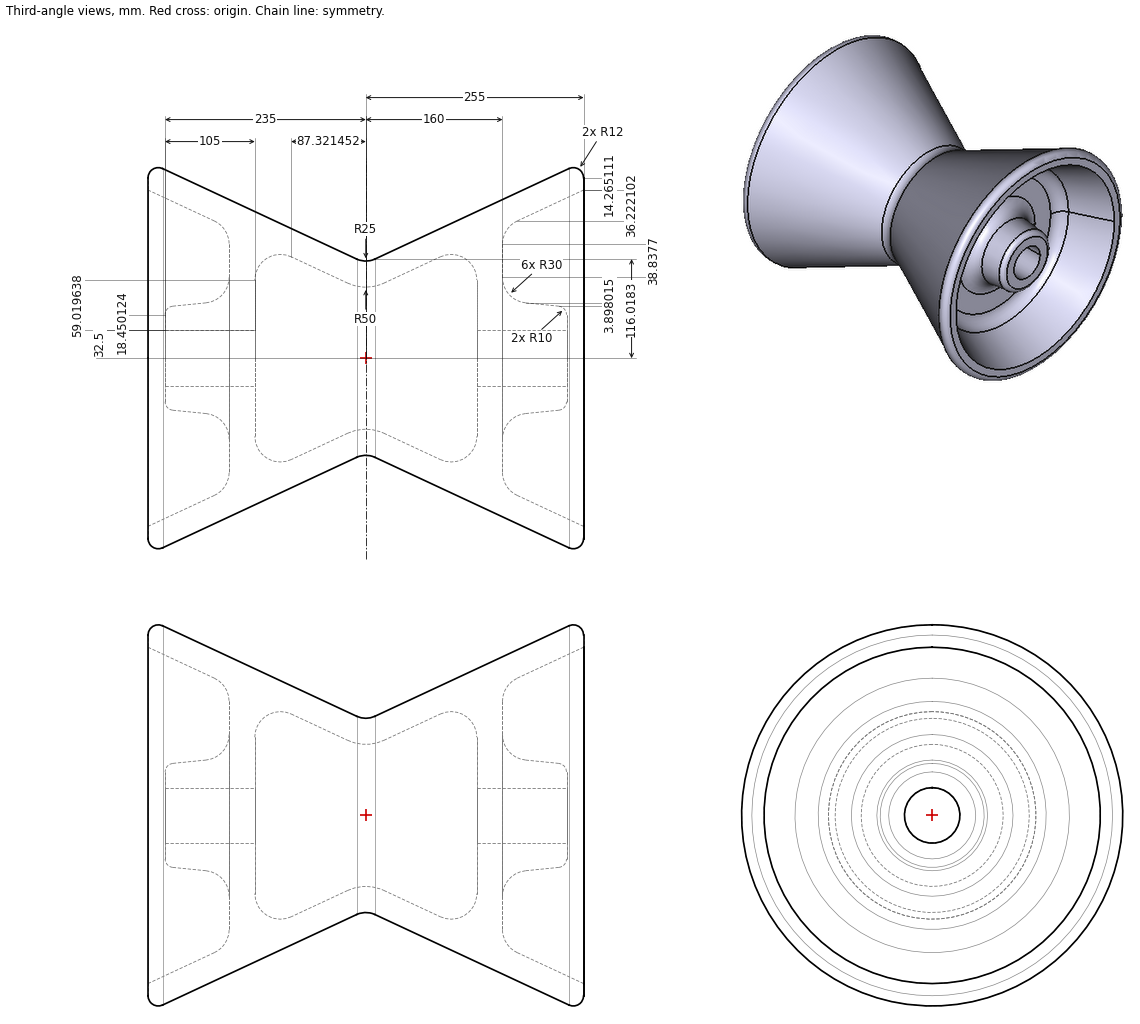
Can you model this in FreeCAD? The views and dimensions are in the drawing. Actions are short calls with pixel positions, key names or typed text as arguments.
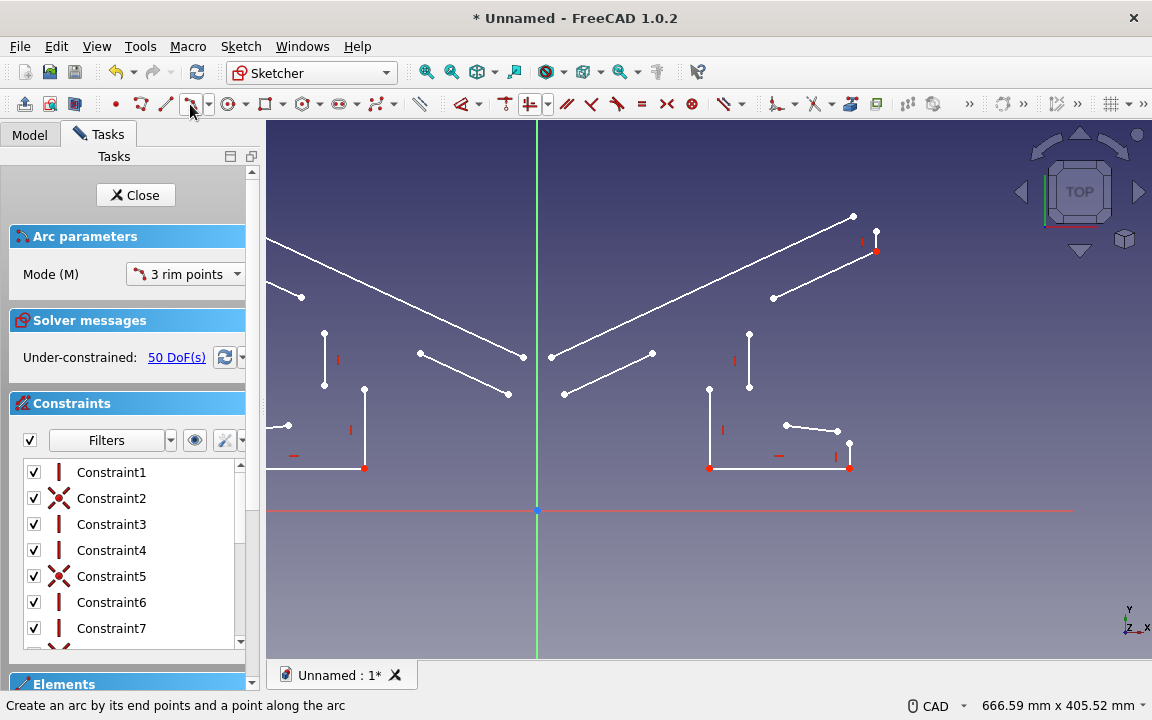
click(787, 426)
click(749, 387)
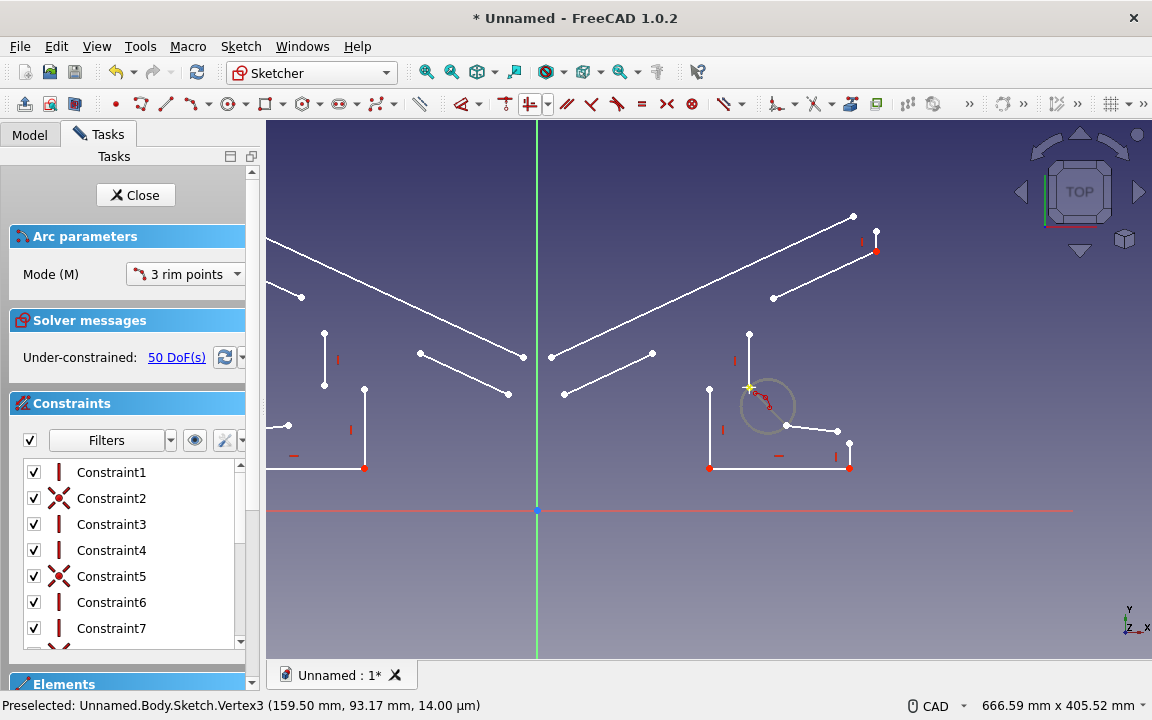
scroll(760, 412, up, 3)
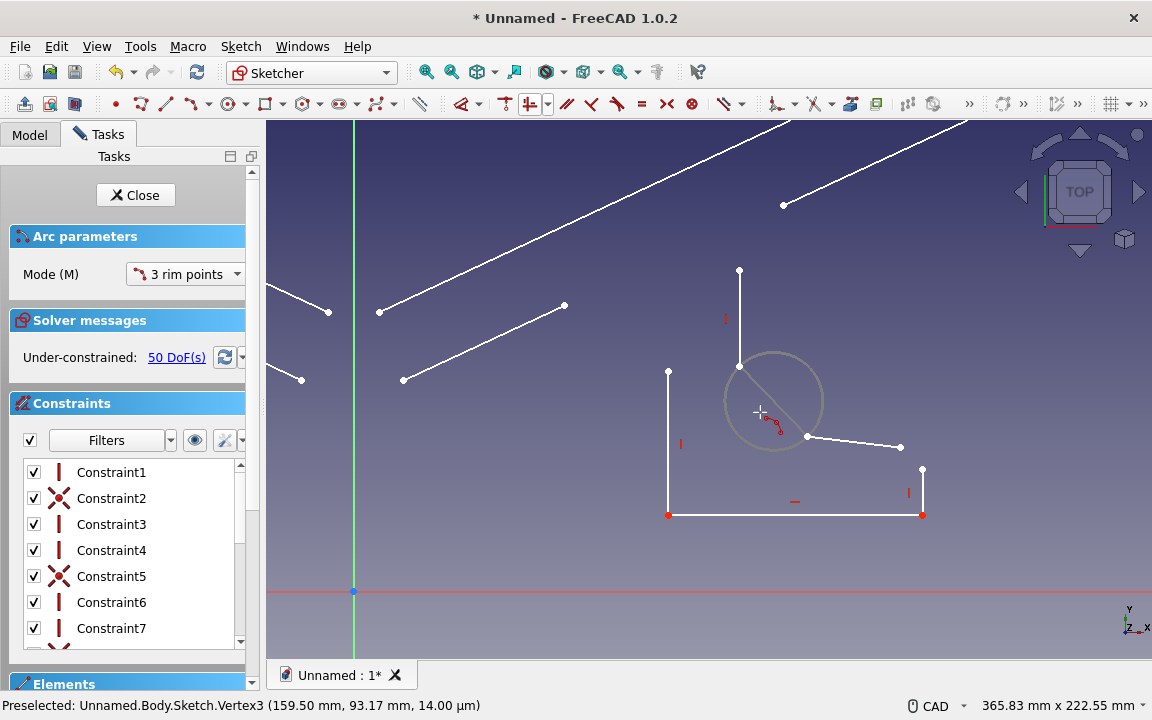
click(760, 411)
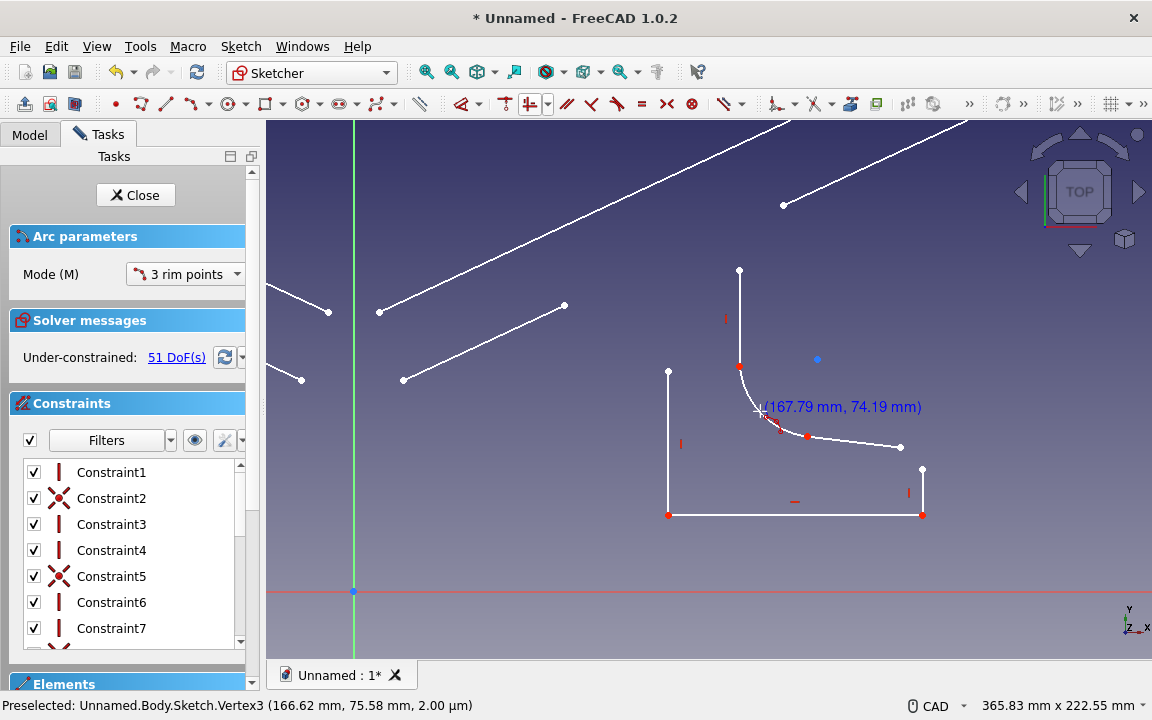
click(740, 271)
click(783, 206)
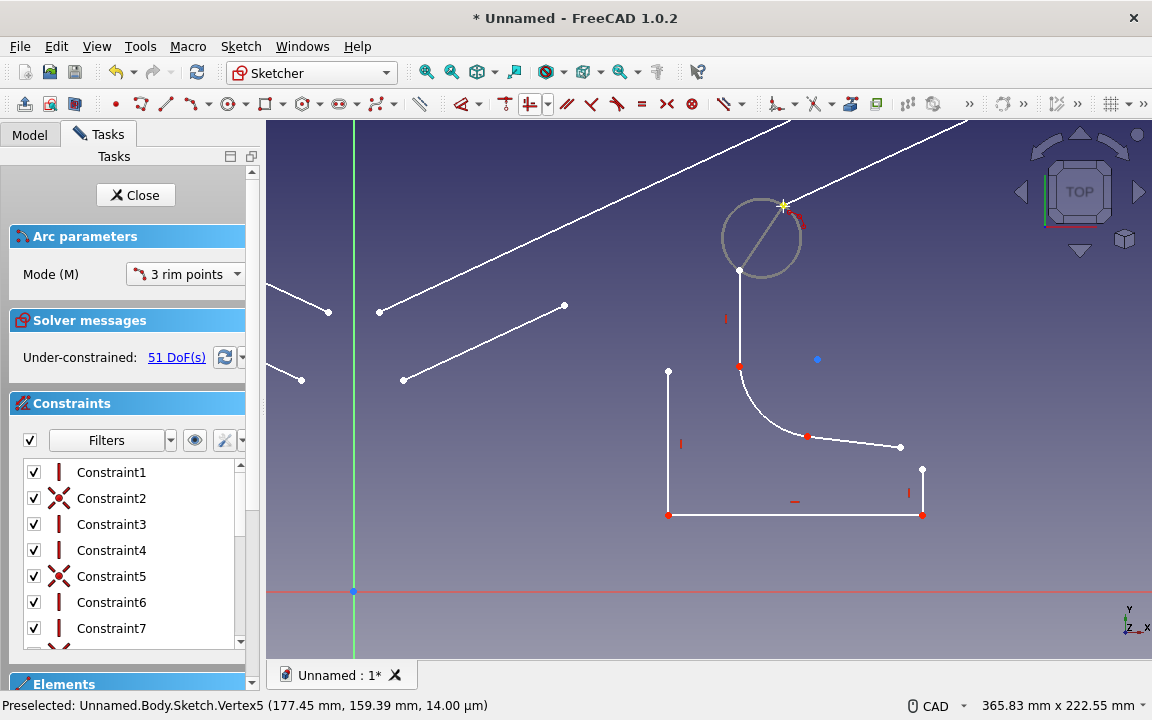
scroll(753, 229, up, 2)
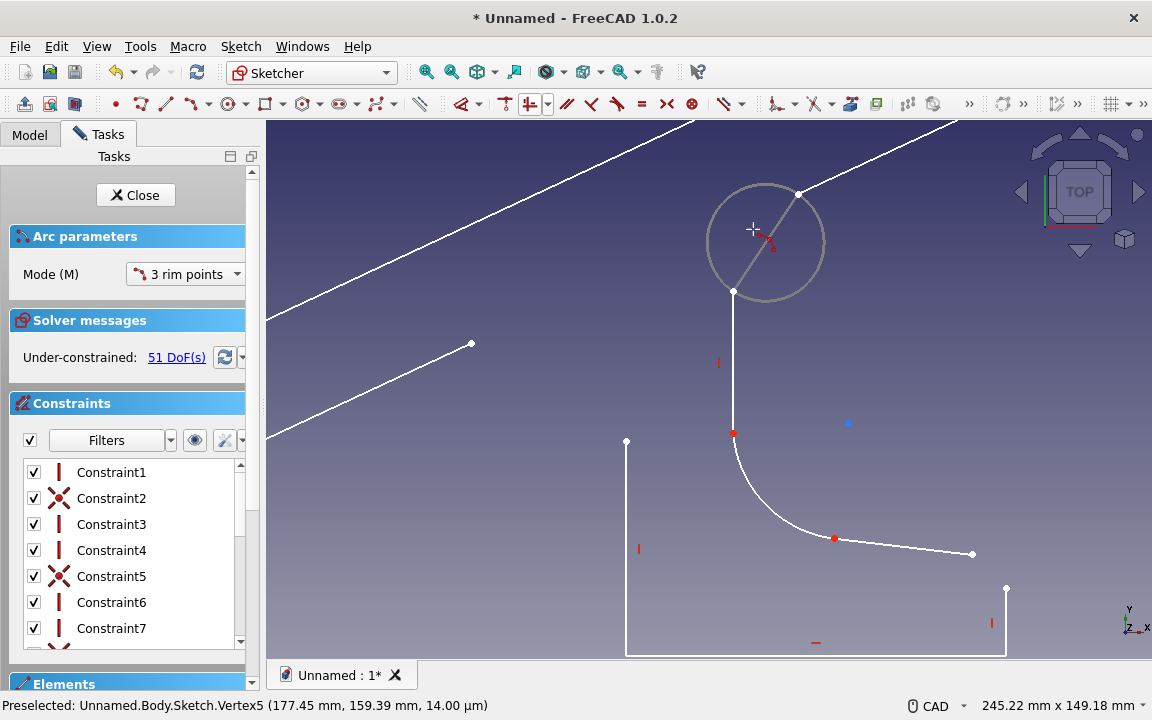
click(752, 229)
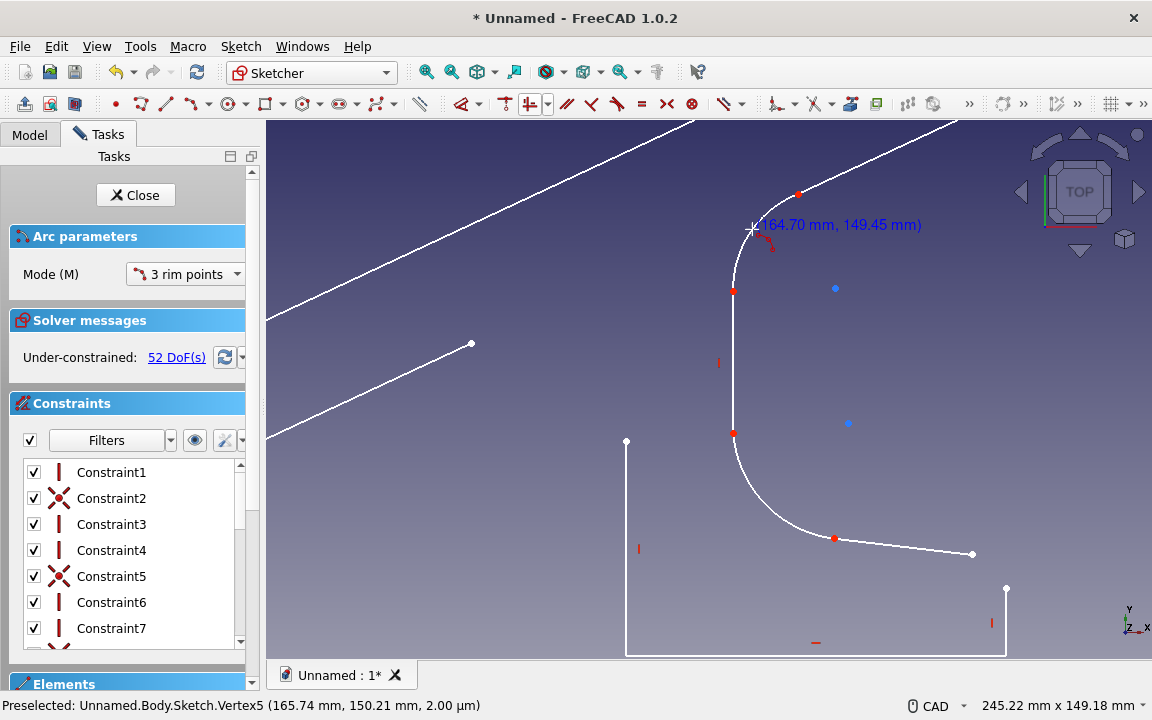
scroll(799, 396, down, 7)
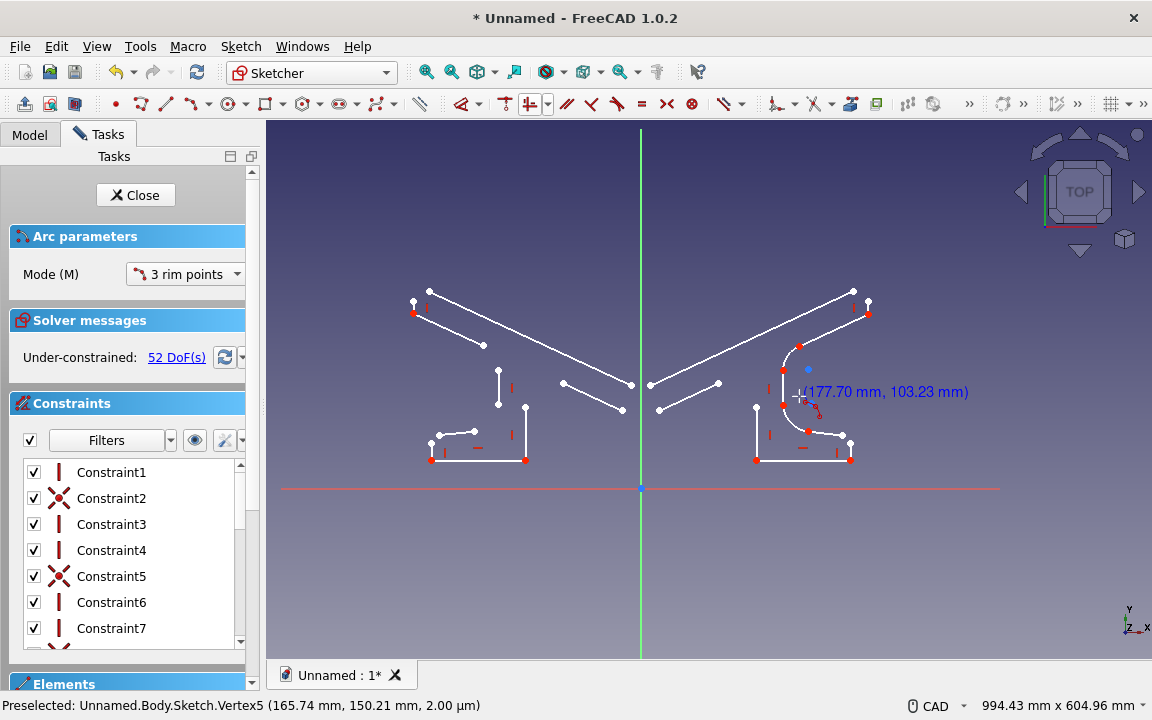
scroll(868, 300, up, 5)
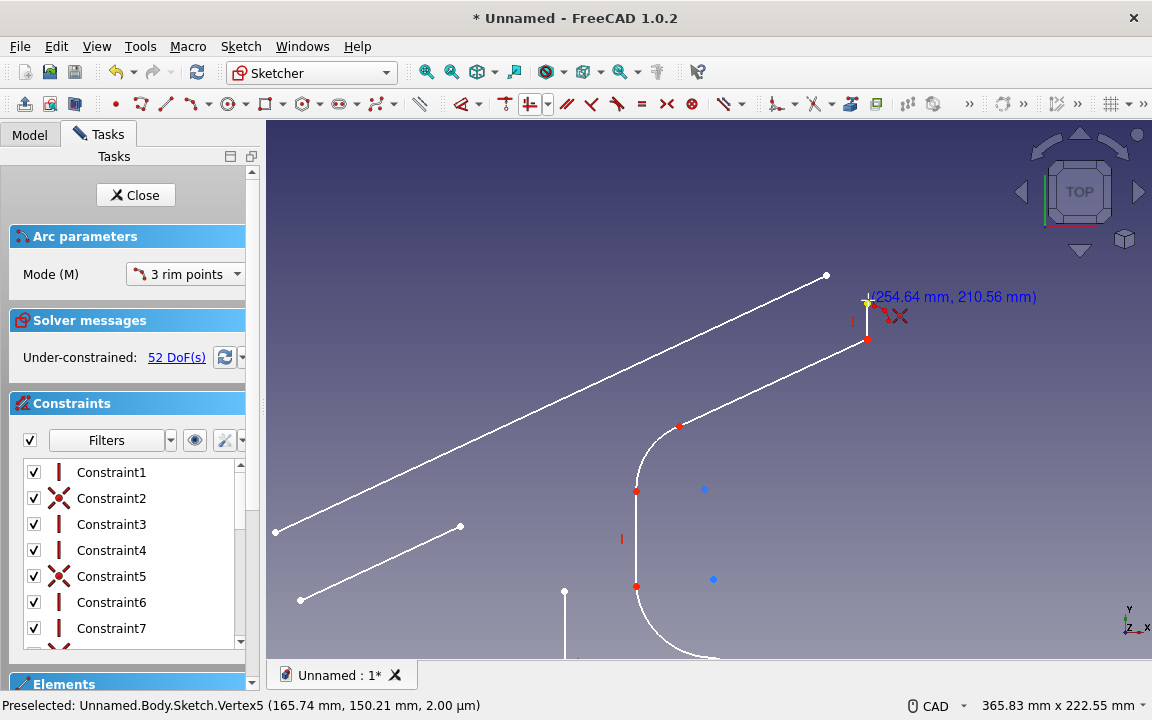
click(867, 303)
click(826, 276)
click(854, 276)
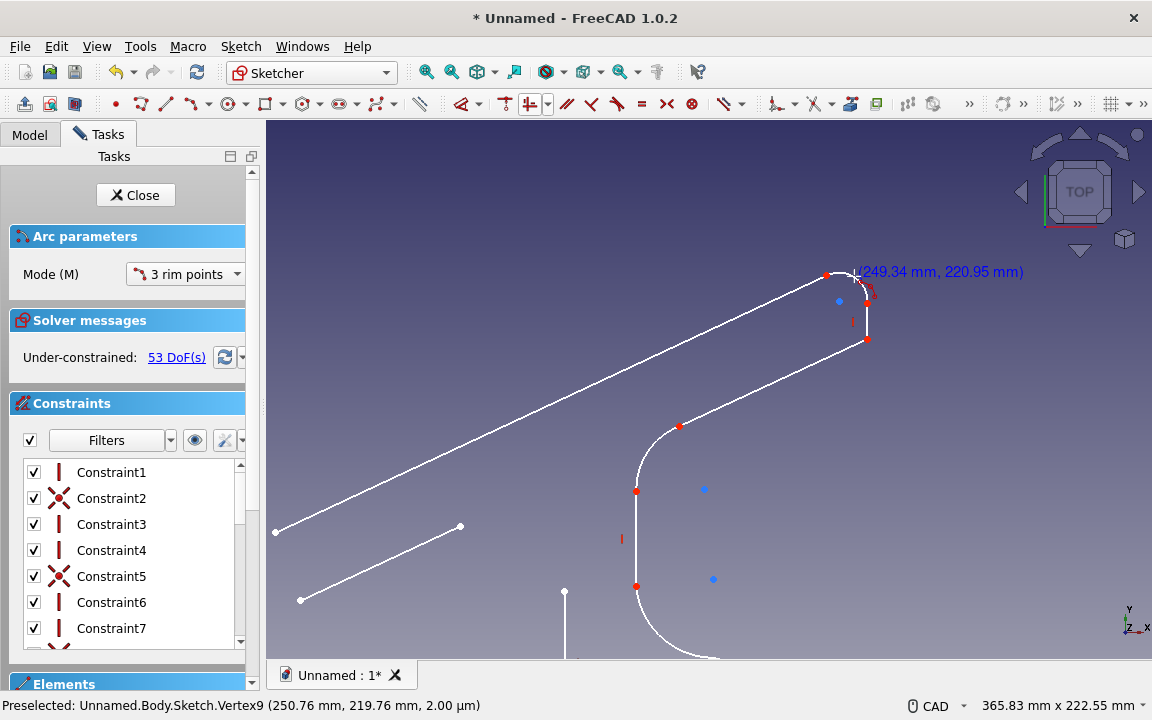
scroll(868, 300, down, 5)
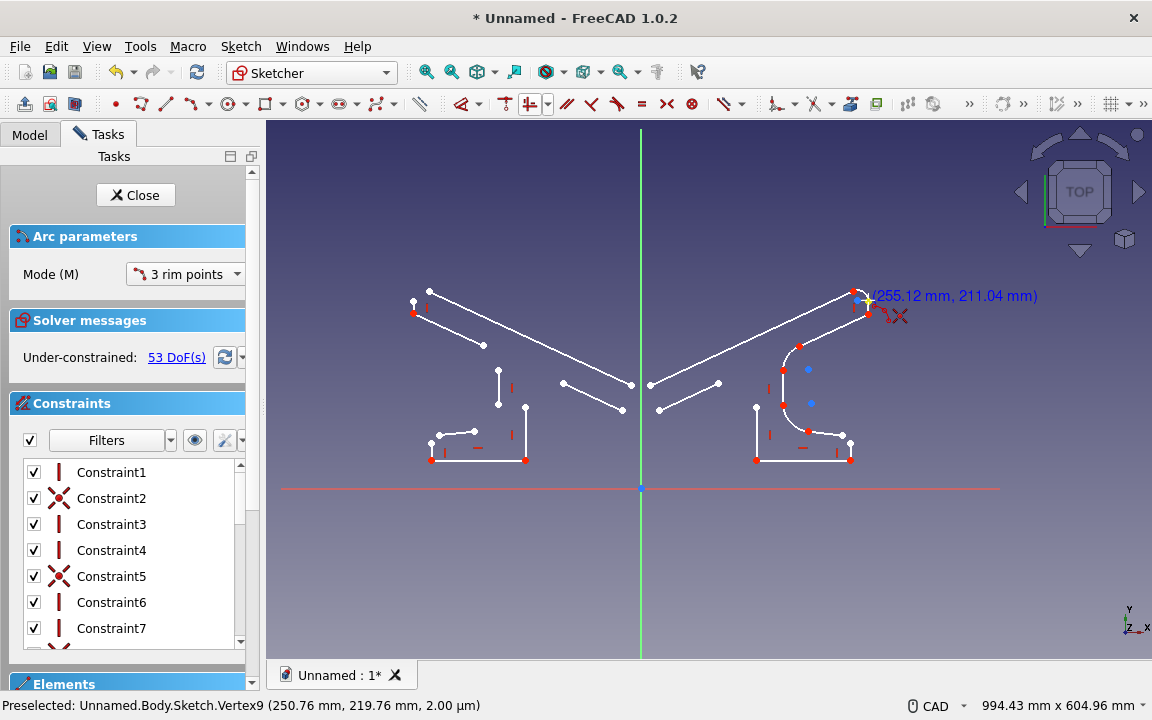
scroll(651, 385, up, 3)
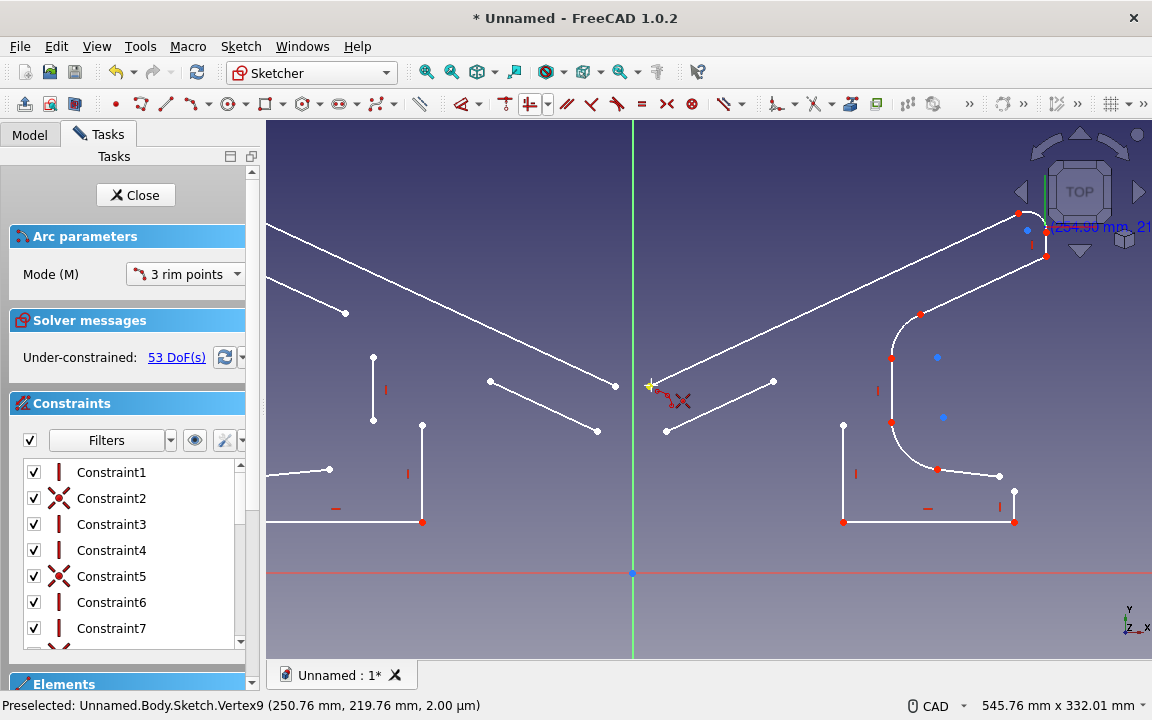
click(650, 386)
click(616, 386)